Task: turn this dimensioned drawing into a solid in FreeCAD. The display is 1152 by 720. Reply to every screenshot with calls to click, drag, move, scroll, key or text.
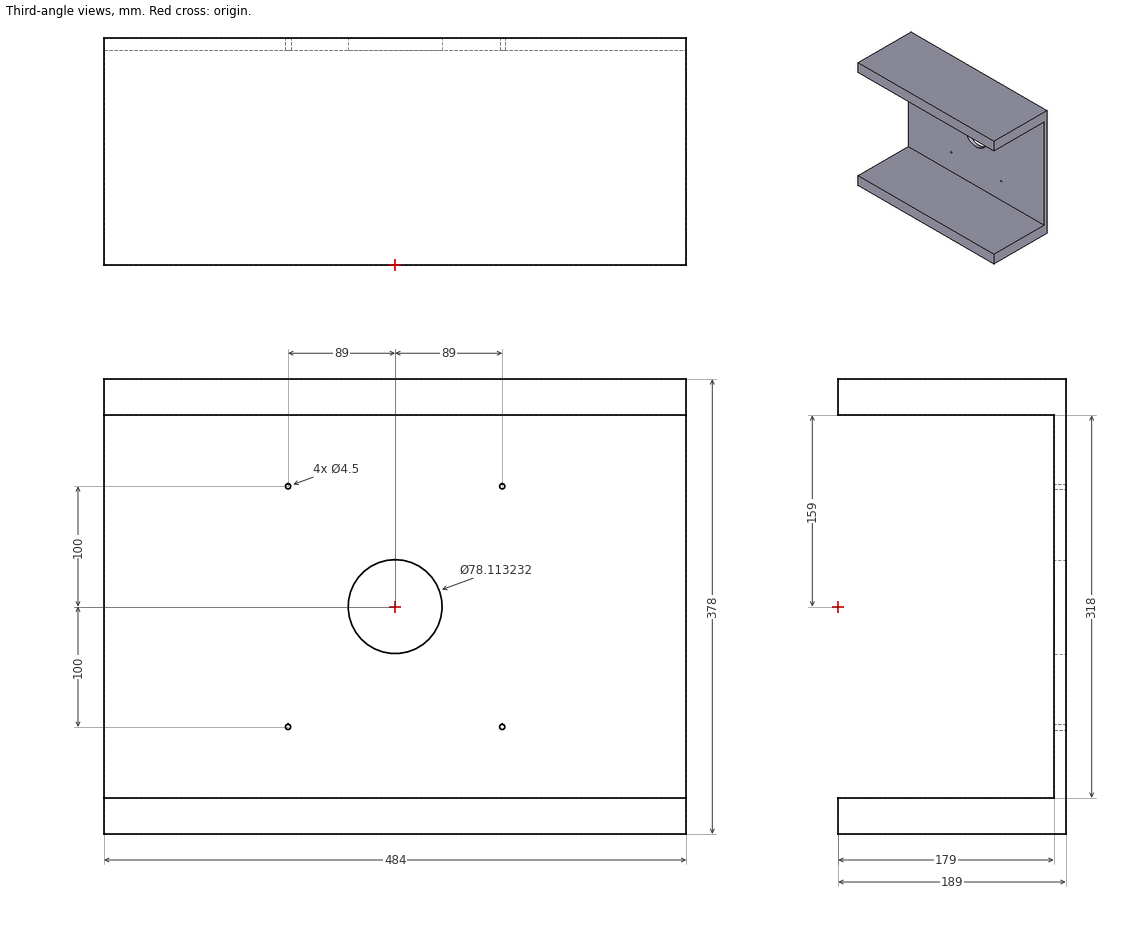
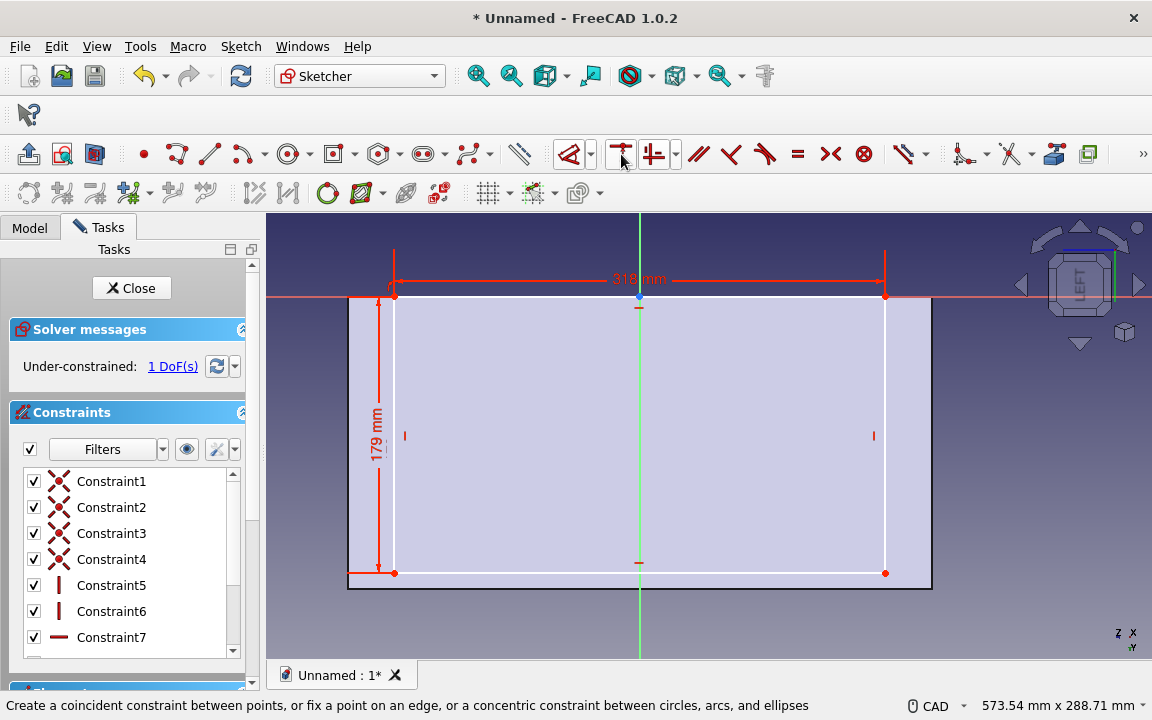
click(568, 154)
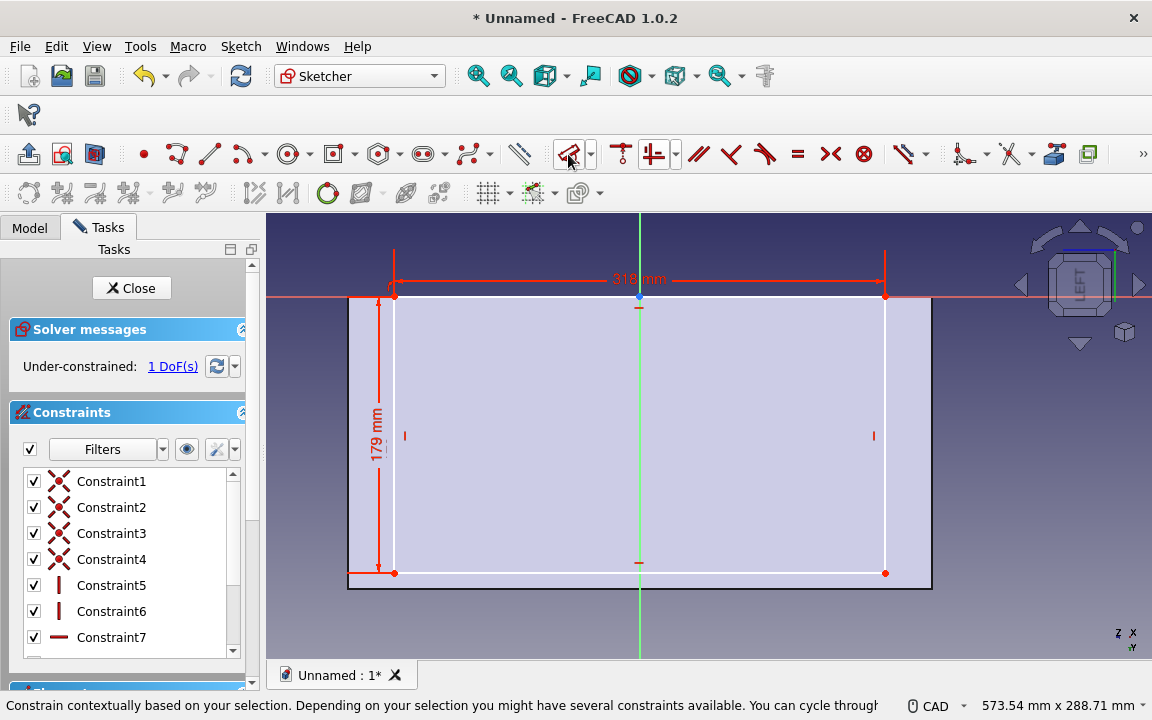
click(394, 297)
click(517, 263)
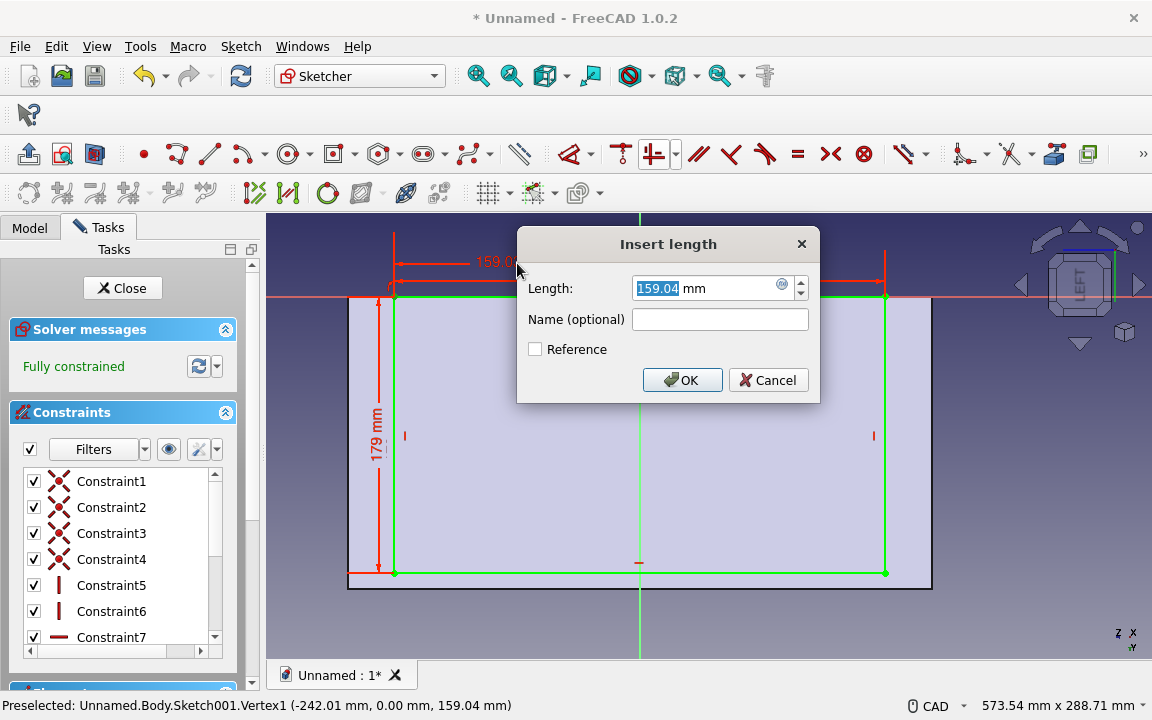
text(159)
key(Return)
key(Escape)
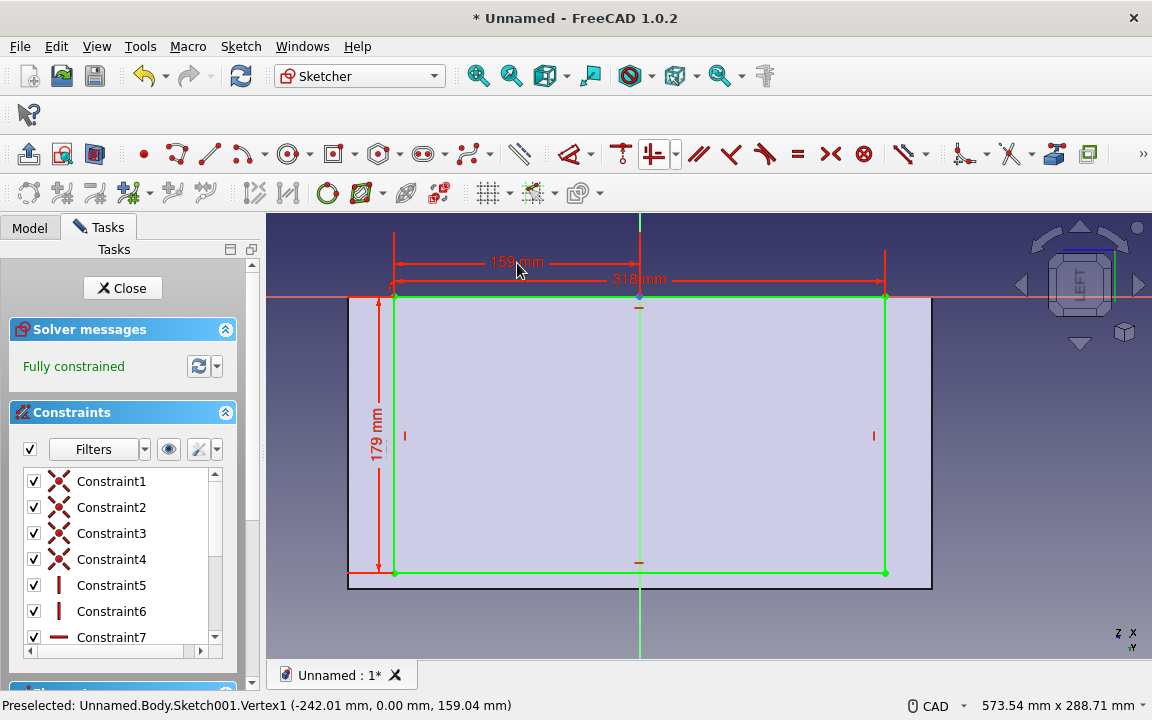
click(123, 288)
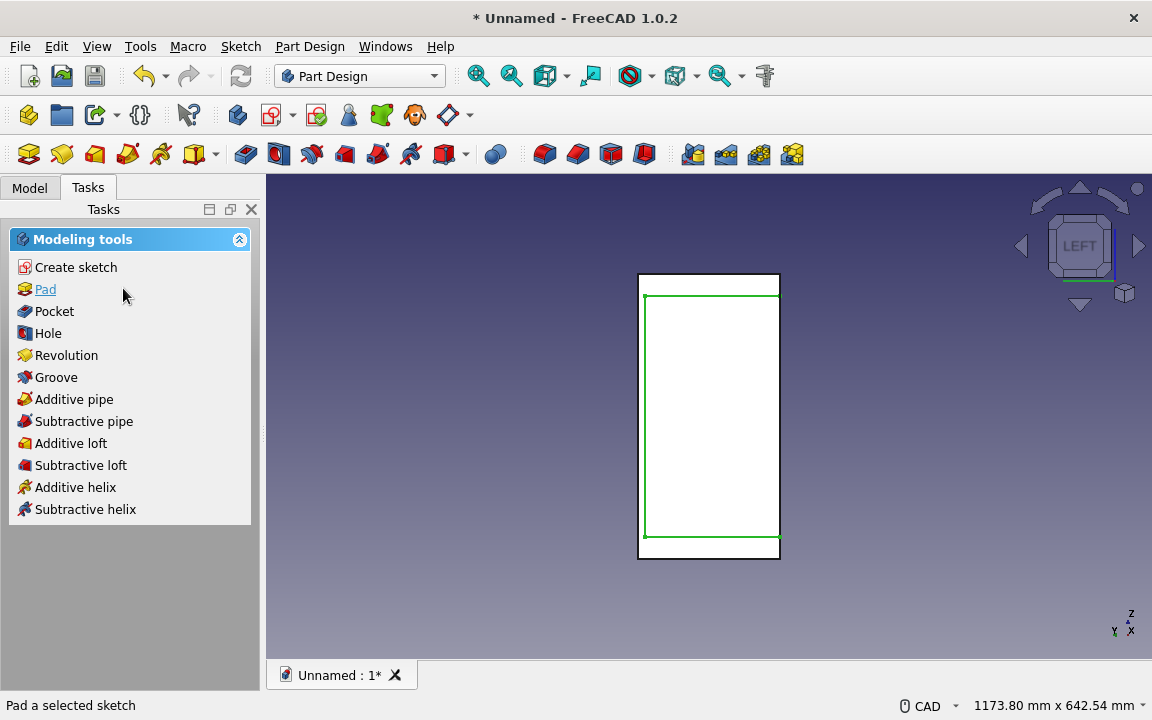
click(246, 154)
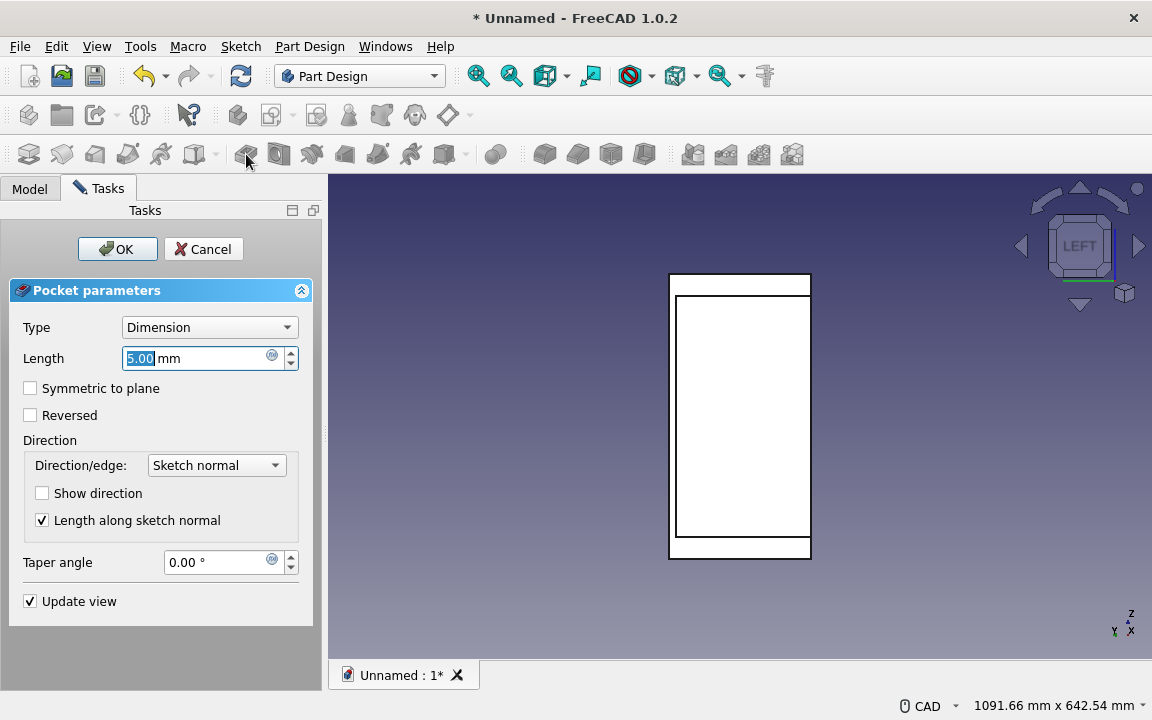
click(210, 328)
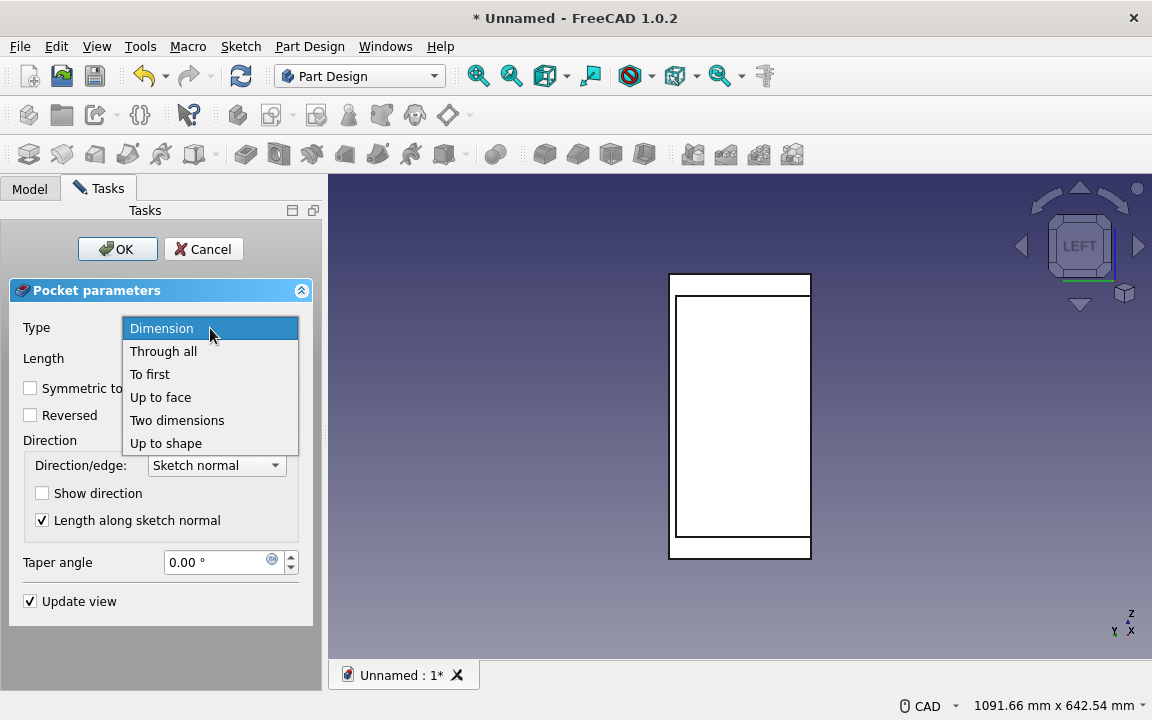
click(208, 352)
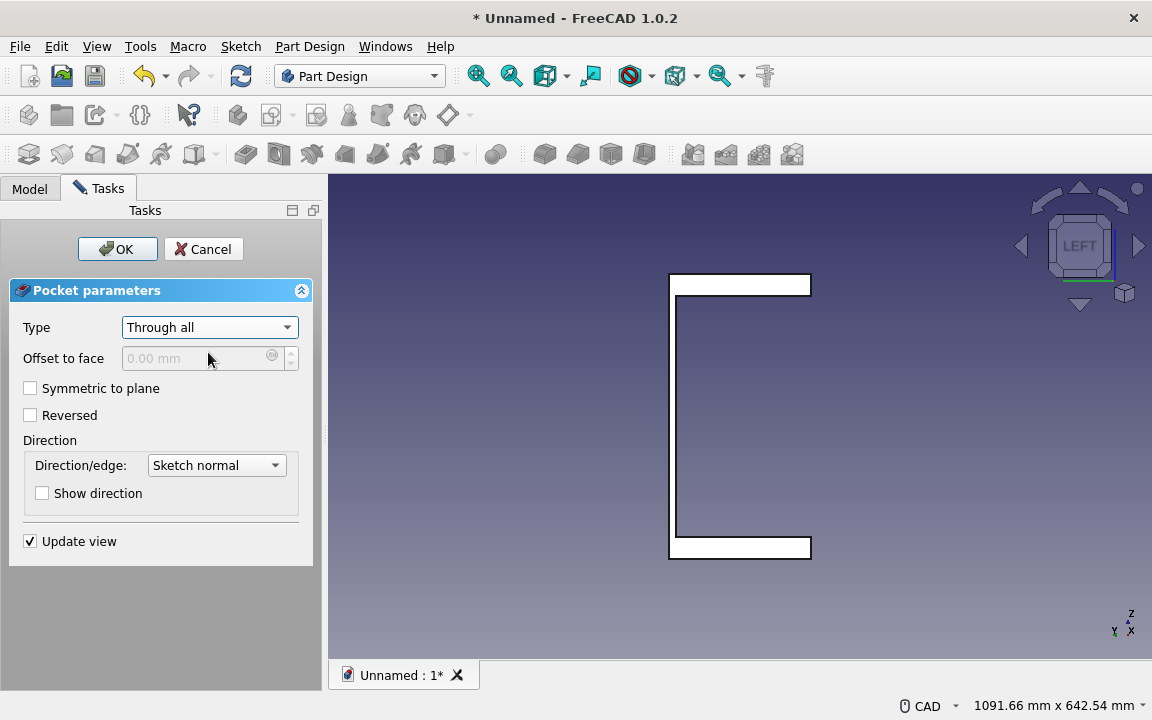
click(118, 249)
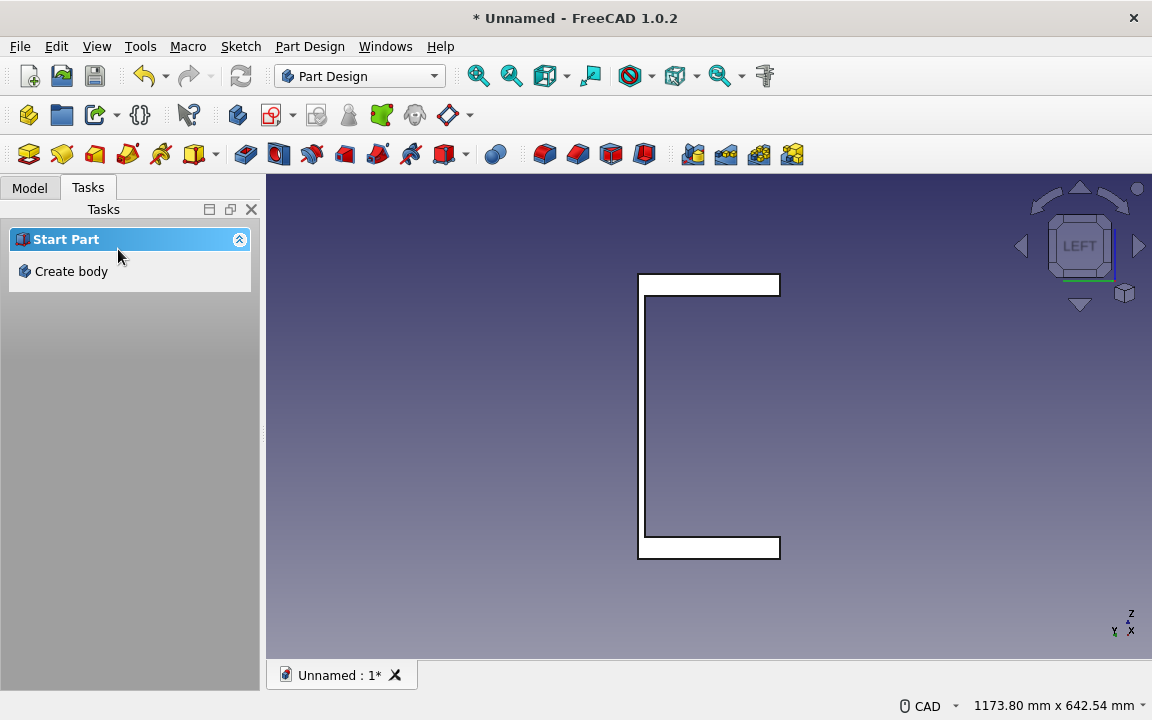
key(4)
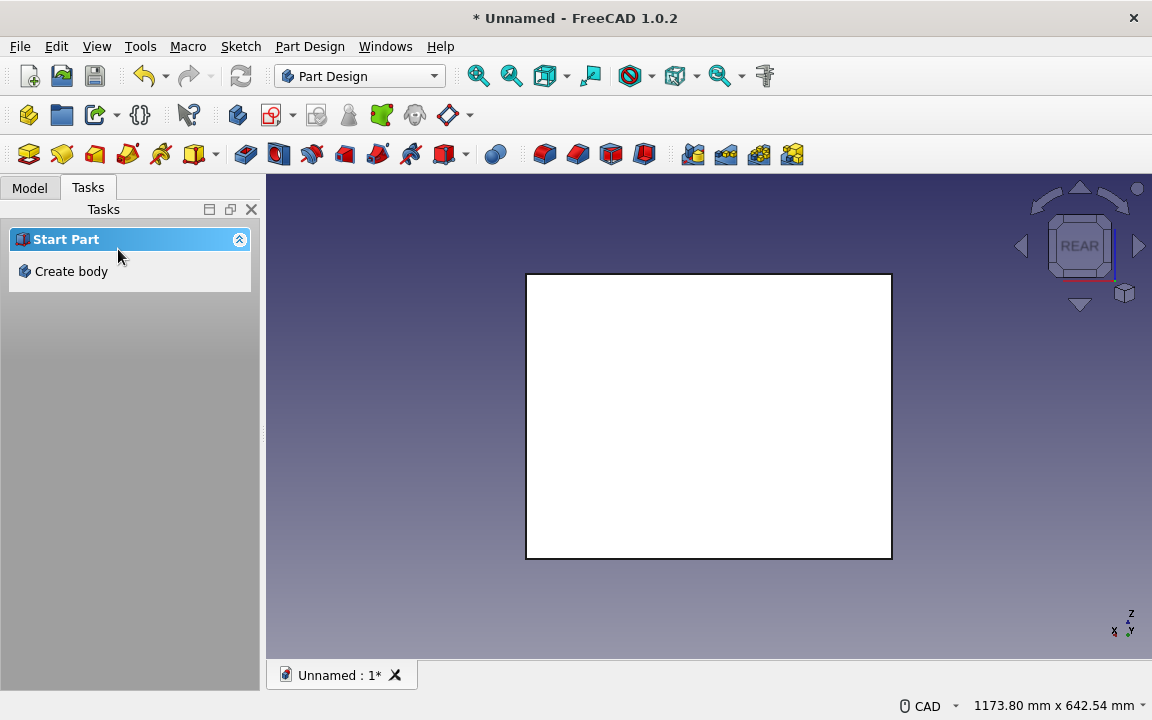
click(709, 416)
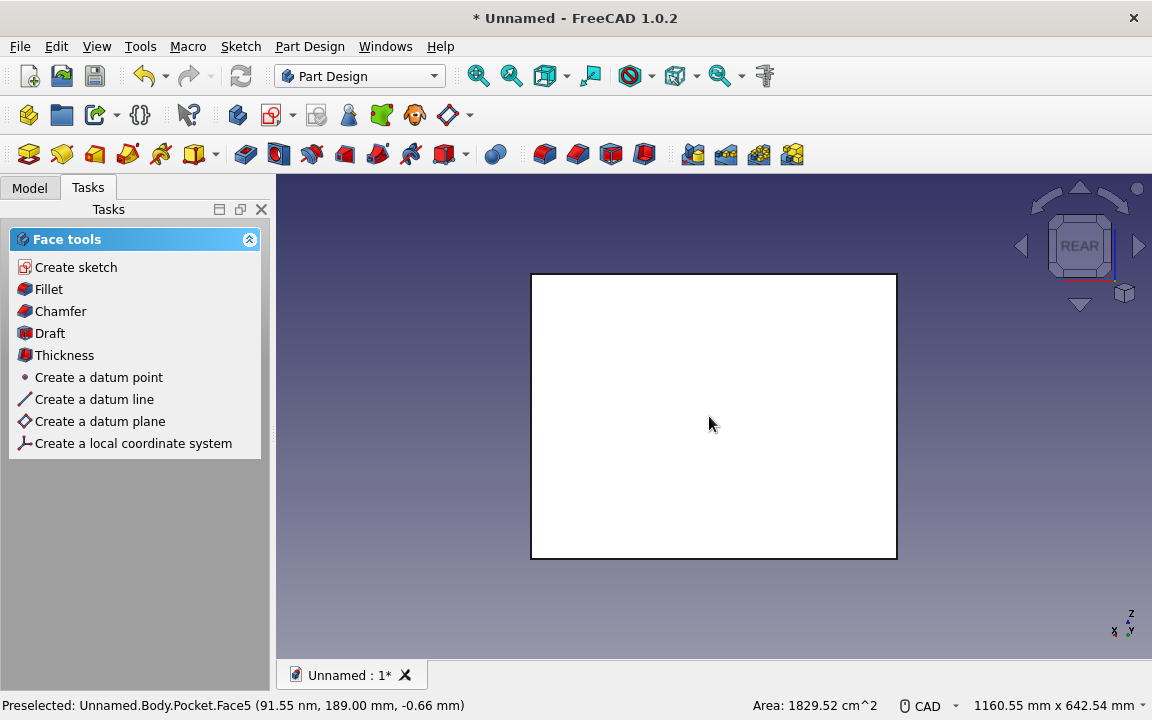
click(270, 116)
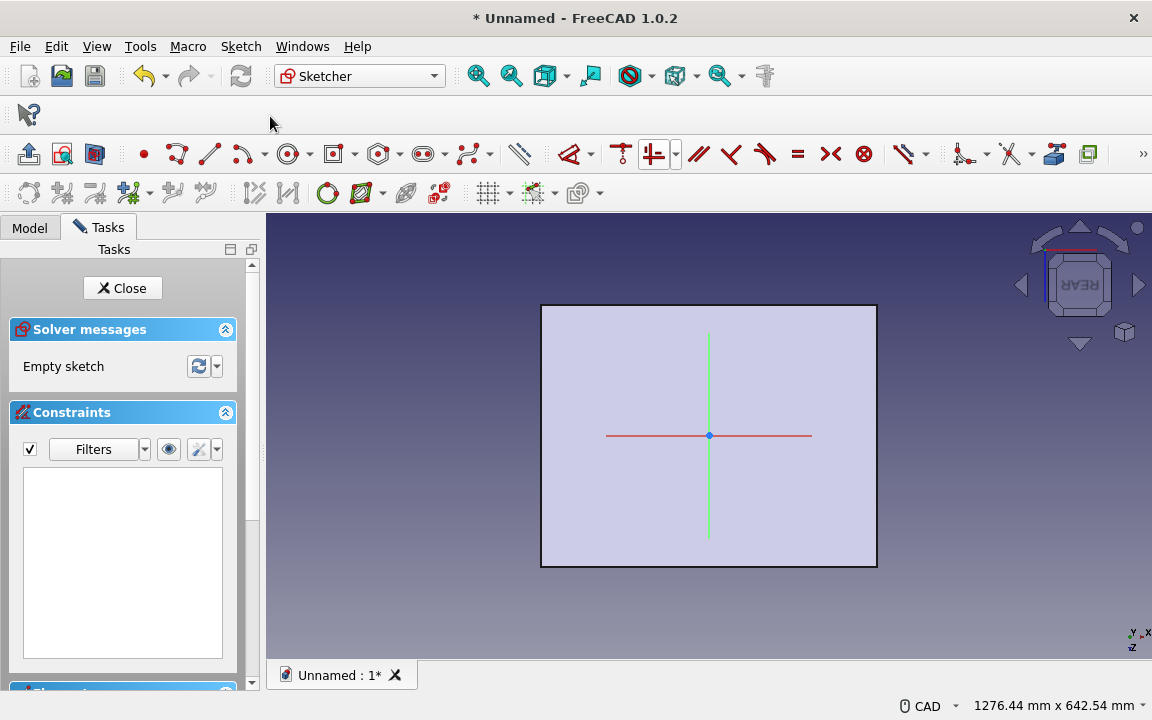
scroll(792, 436, up, 3)